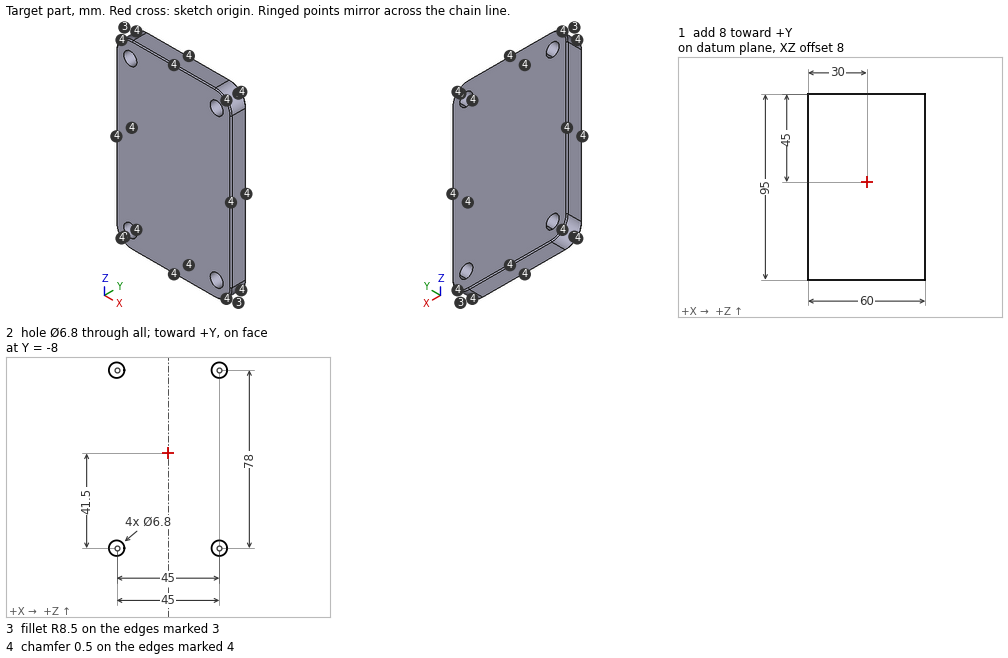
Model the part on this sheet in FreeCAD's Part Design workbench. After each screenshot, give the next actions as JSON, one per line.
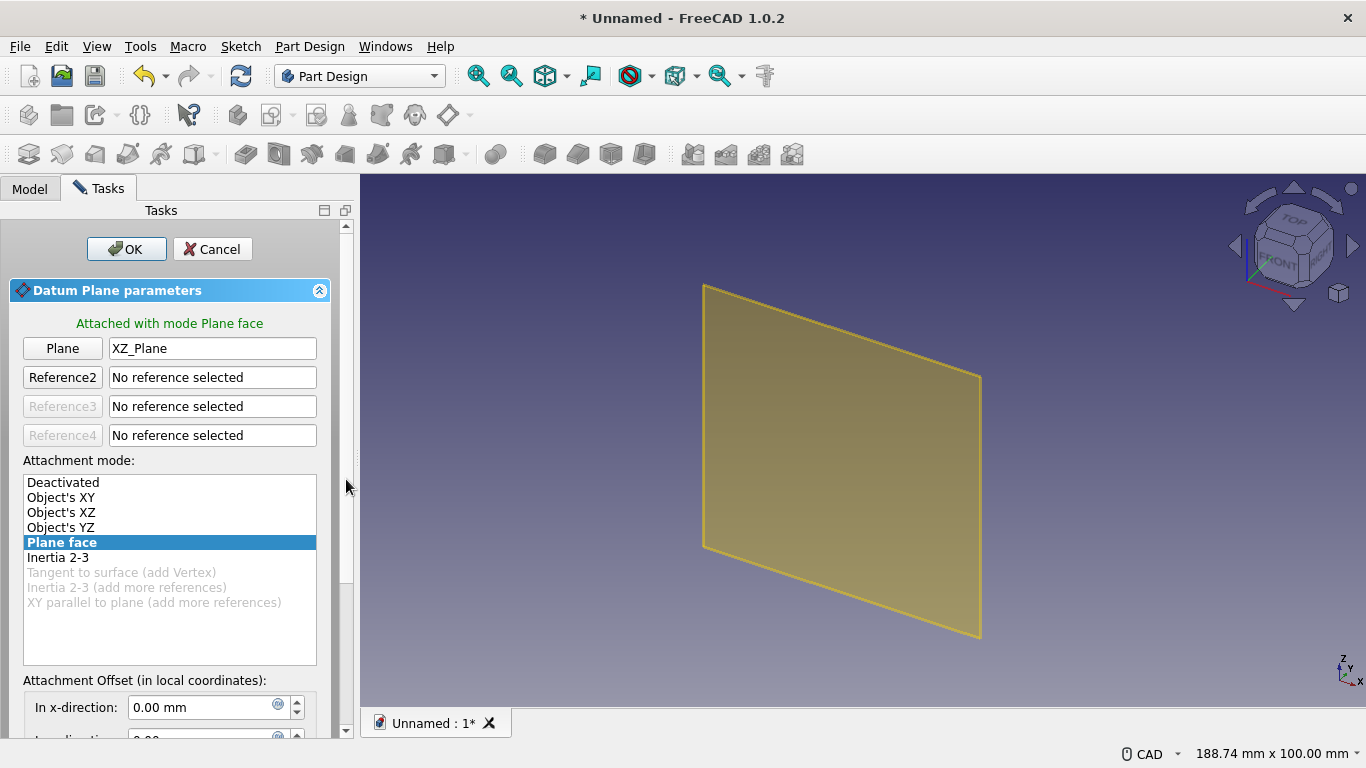
{"action": "left_click", "coordinate": [127, 249]}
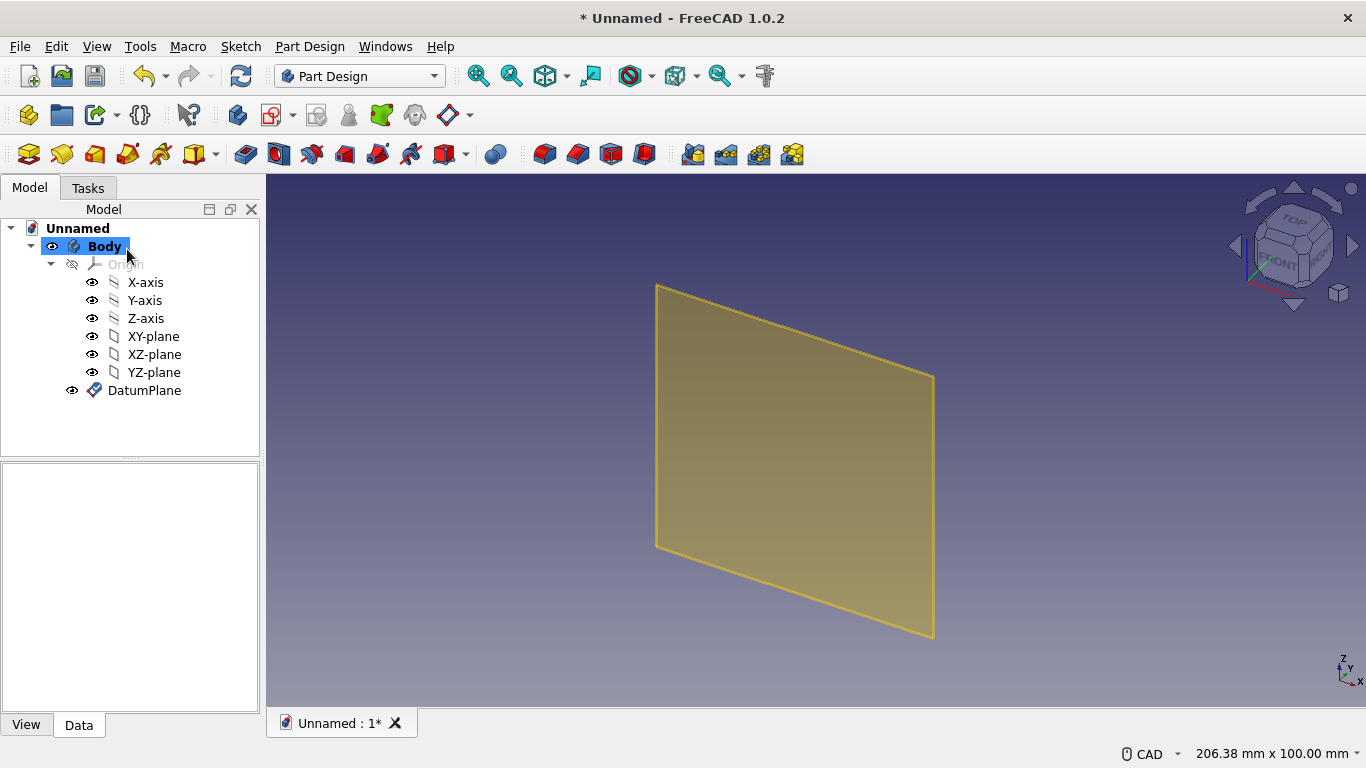
{"action": "left_click", "coordinate": [117, 390]}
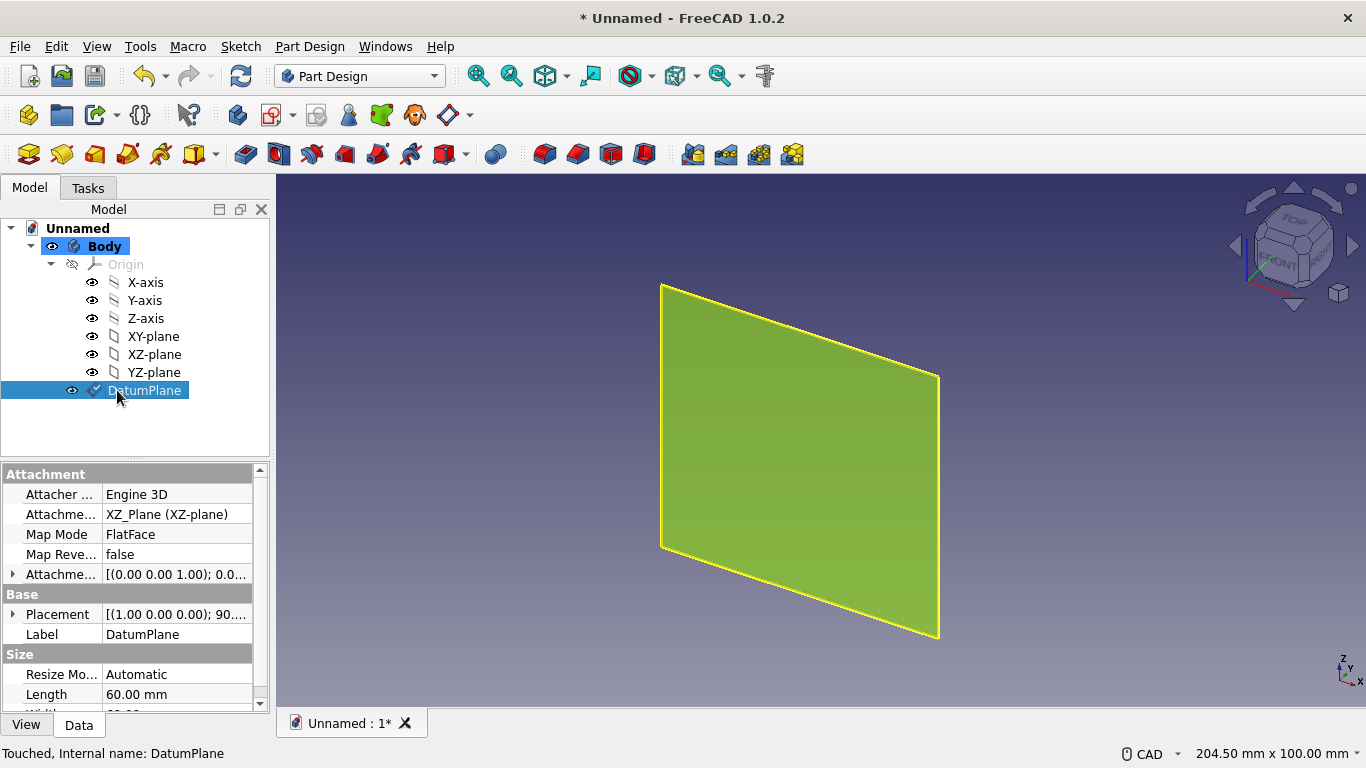
{"action": "left_click", "coordinate": [270, 116]}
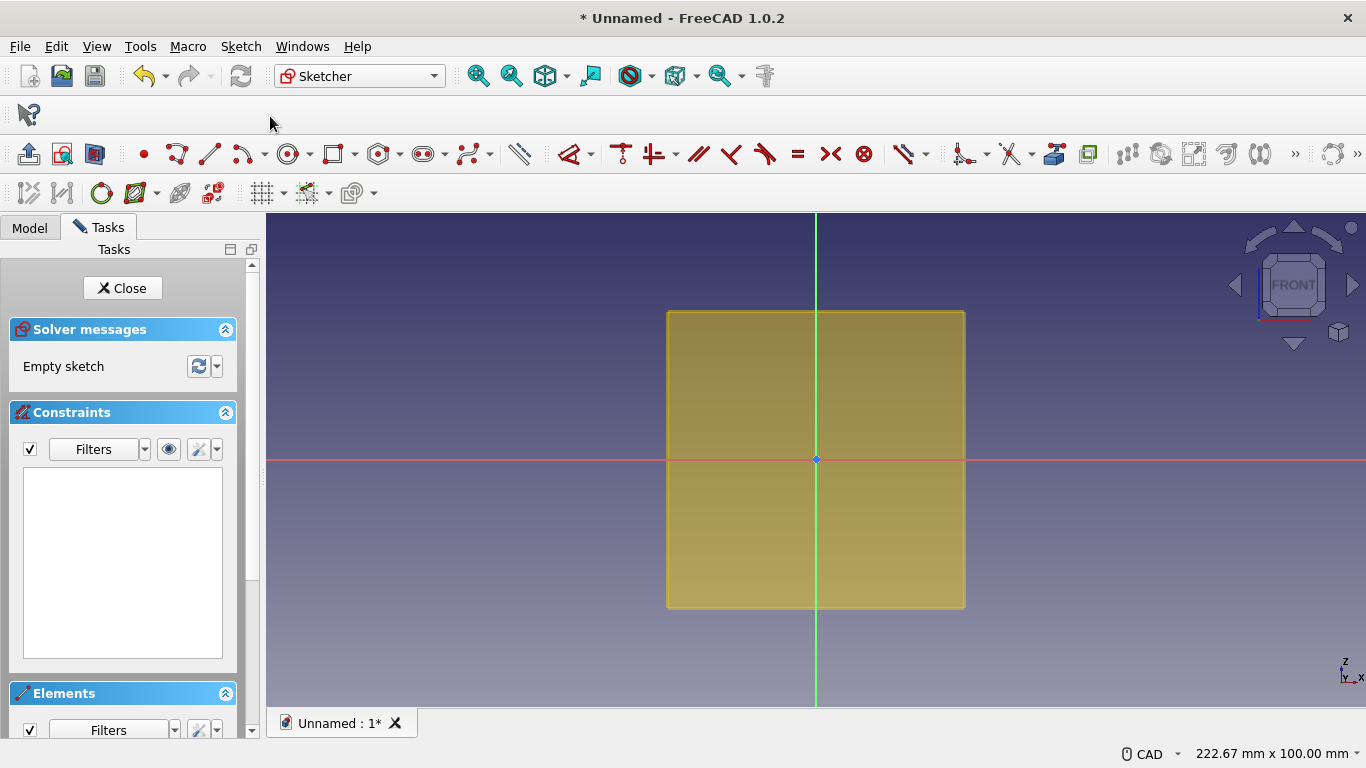
{"action": "scroll", "coordinate": [608, 435], "scroll_direction": "down", "scroll_amount": 2}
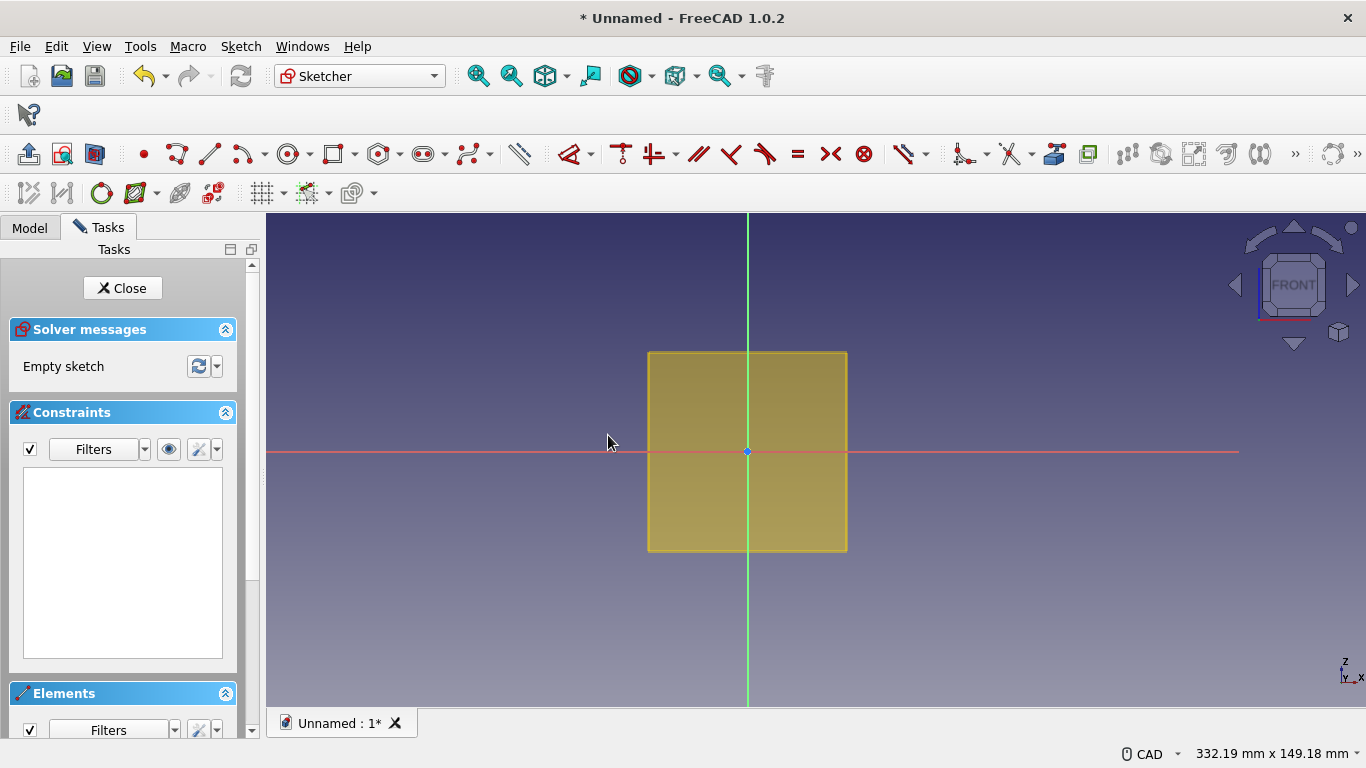
{"action": "left_click", "coordinate": [332, 154]}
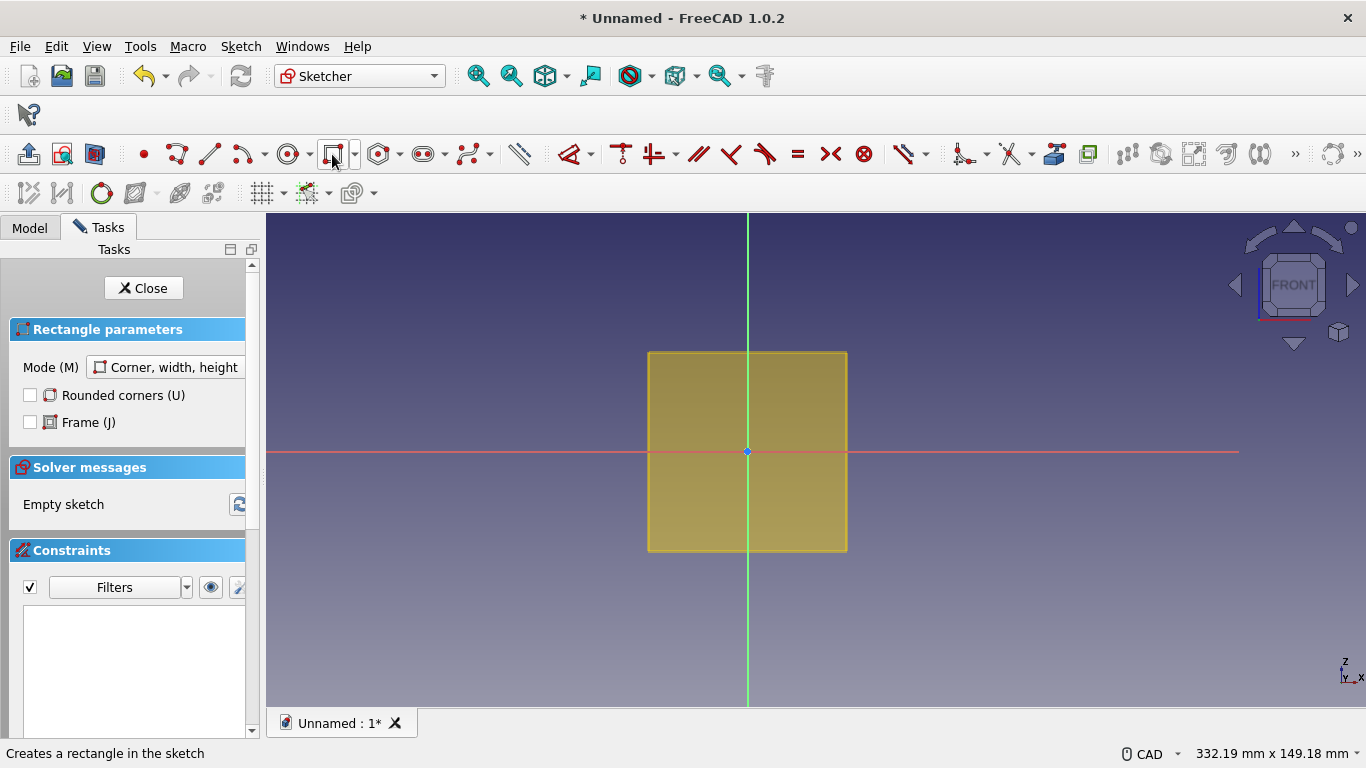
{"action": "left_click", "coordinate": [648, 303]}
{"action": "left_click", "coordinate": [847, 617]}
{"action": "key", "text": "Escape"}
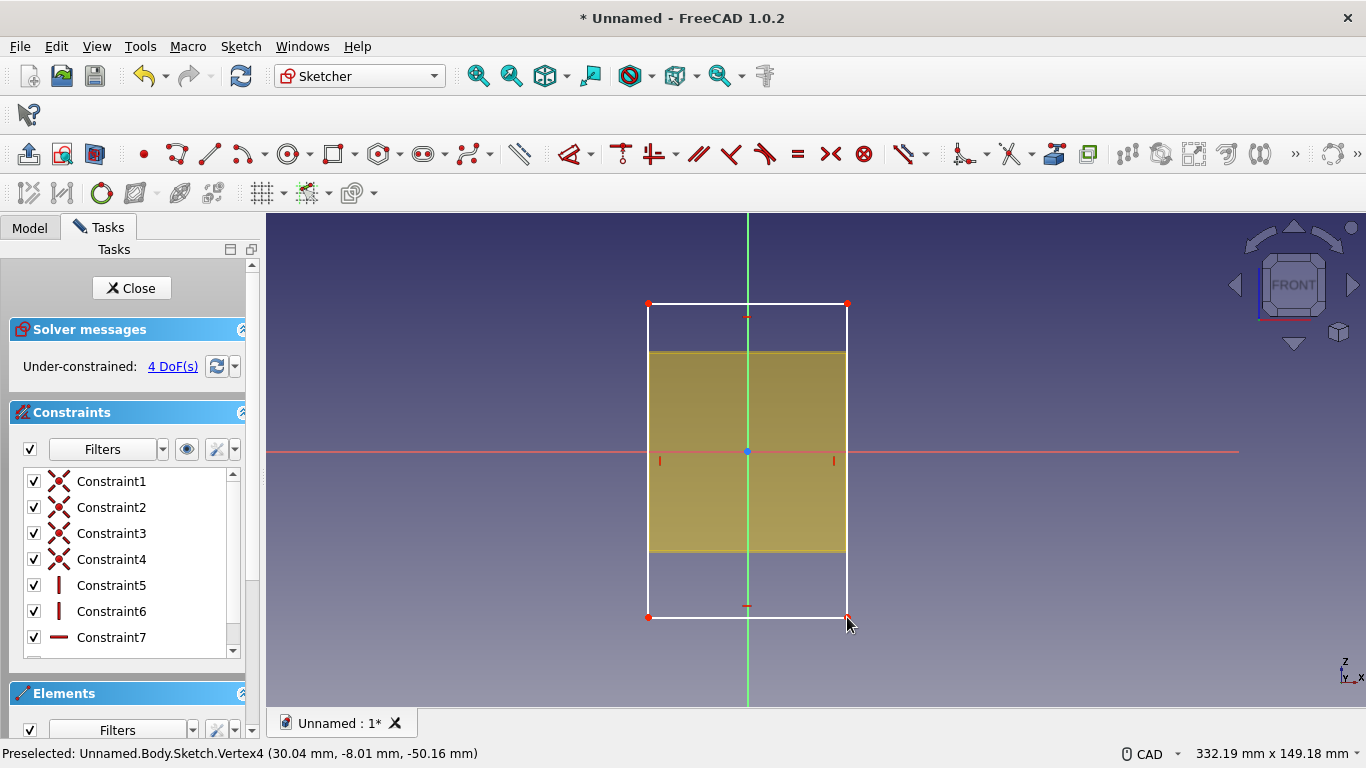
{"action": "left_click", "coordinate": [568, 154]}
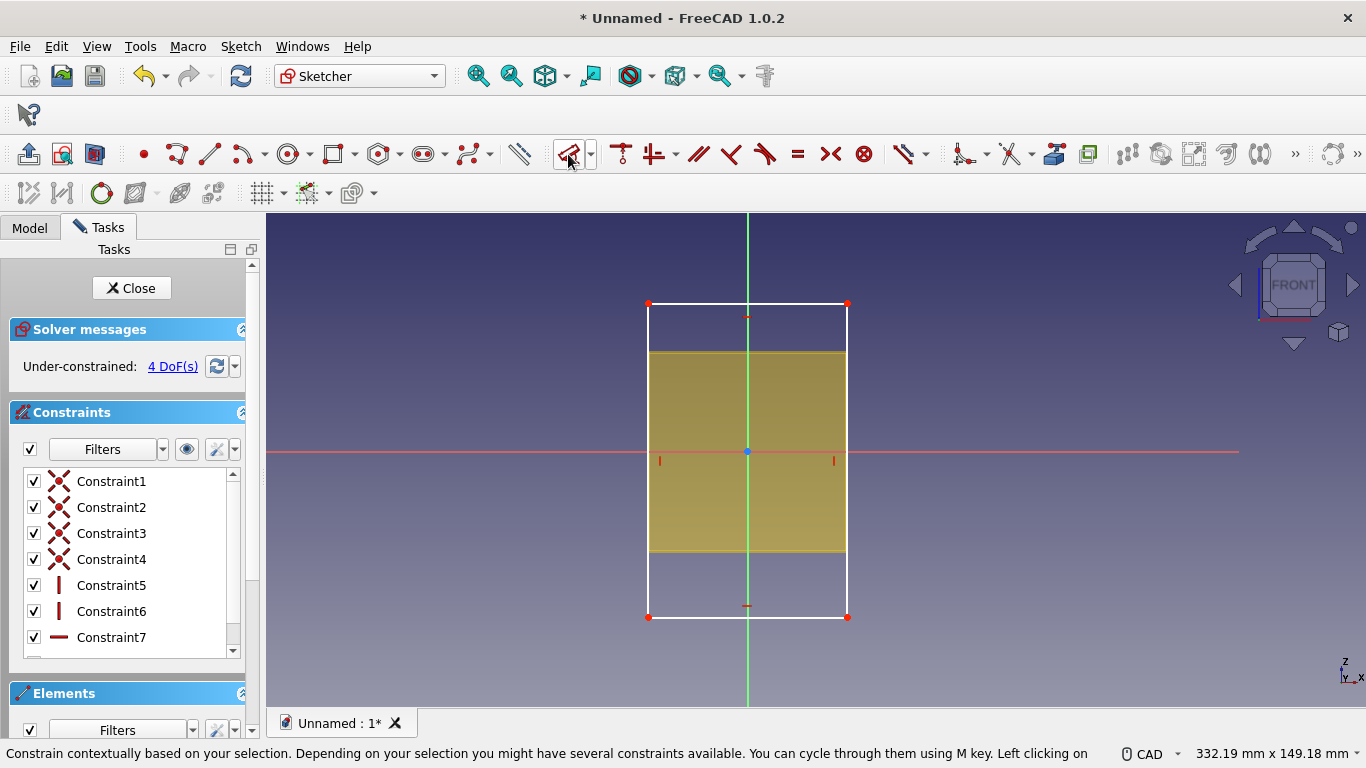
{"action": "left_click", "coordinate": [648, 398]}
{"action": "left_click", "coordinate": [614, 389]}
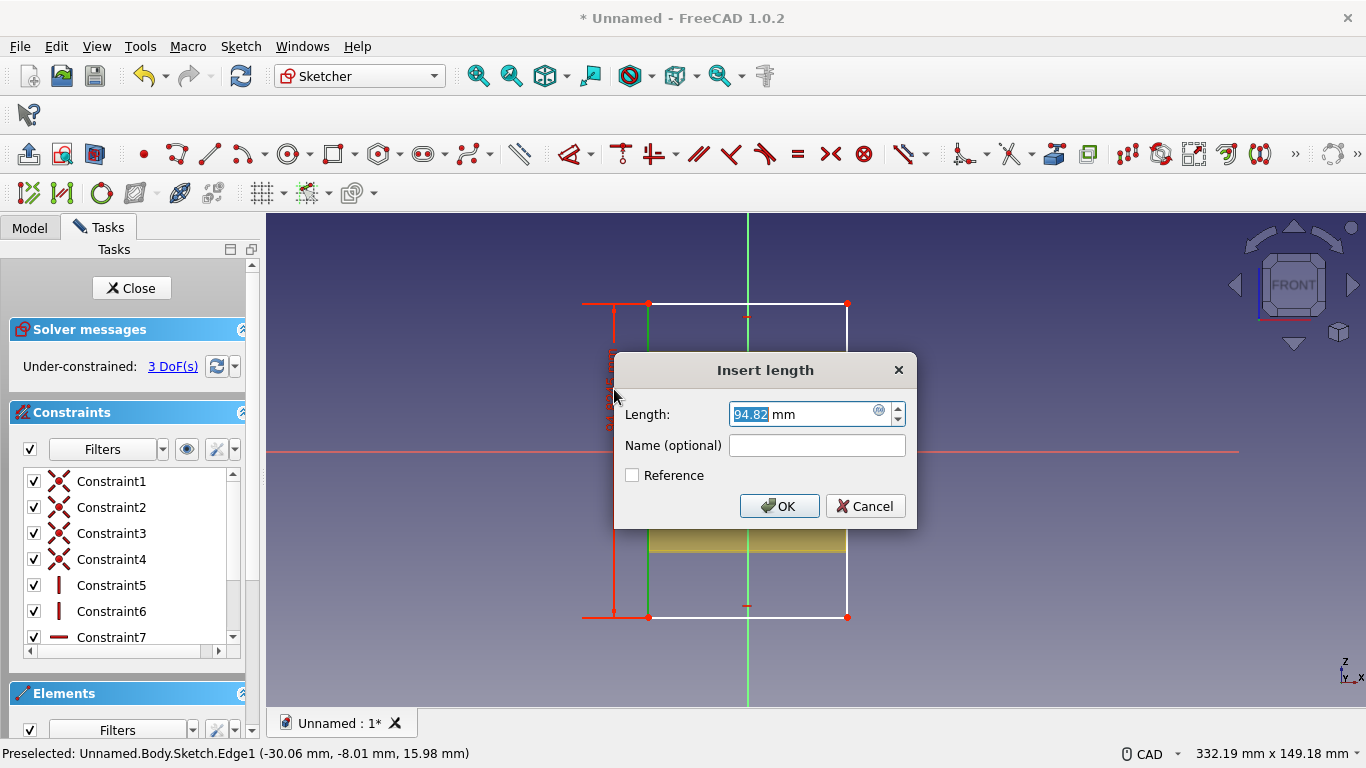
{"action": "type", "text": "95"}
{"action": "key", "text": "Return"}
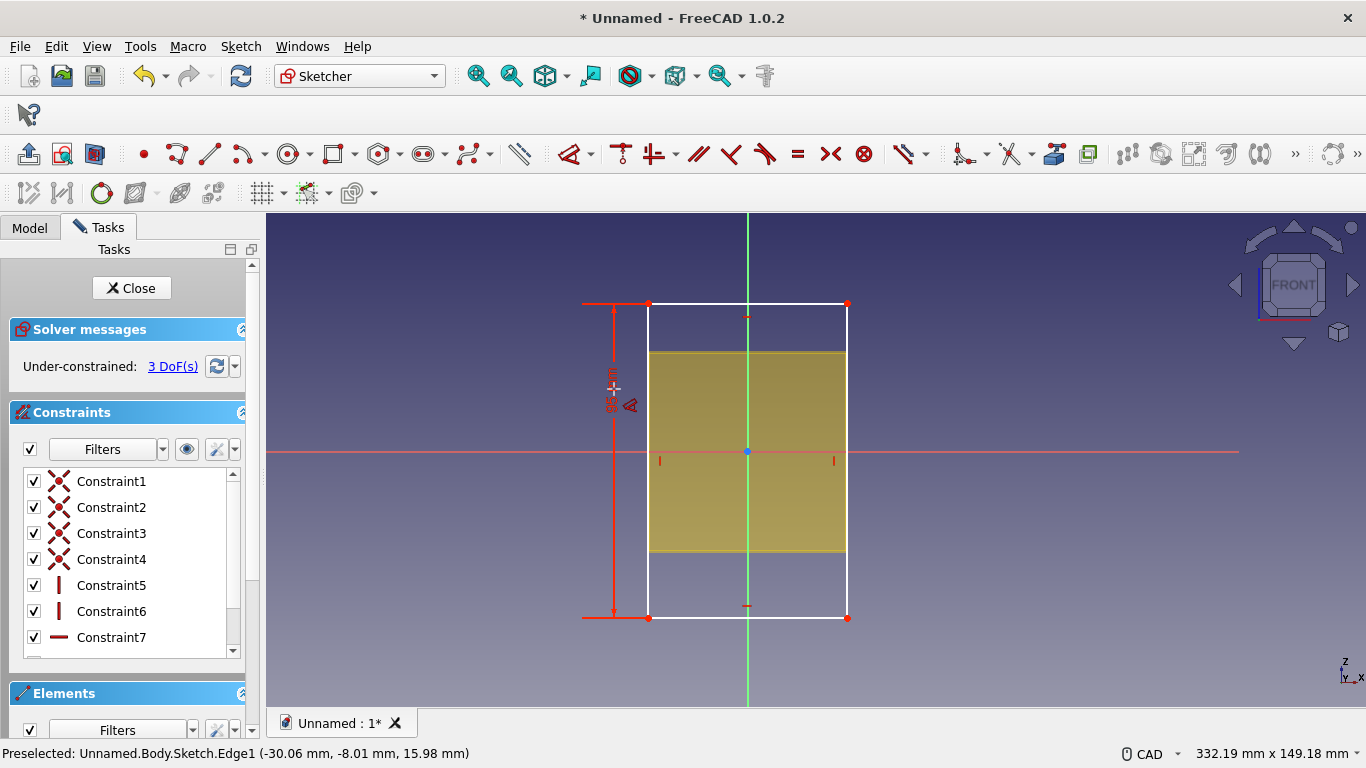
{"action": "left_click", "coordinate": [708, 618]}
{"action": "left_click", "coordinate": [702, 652]}